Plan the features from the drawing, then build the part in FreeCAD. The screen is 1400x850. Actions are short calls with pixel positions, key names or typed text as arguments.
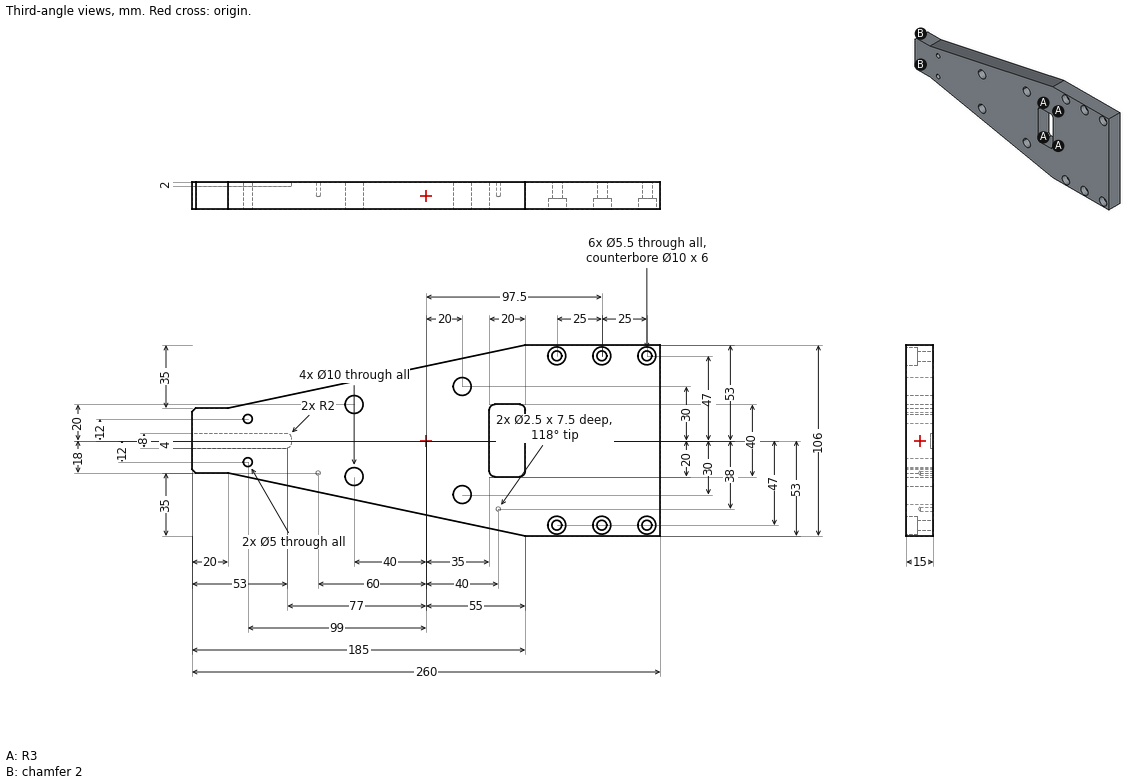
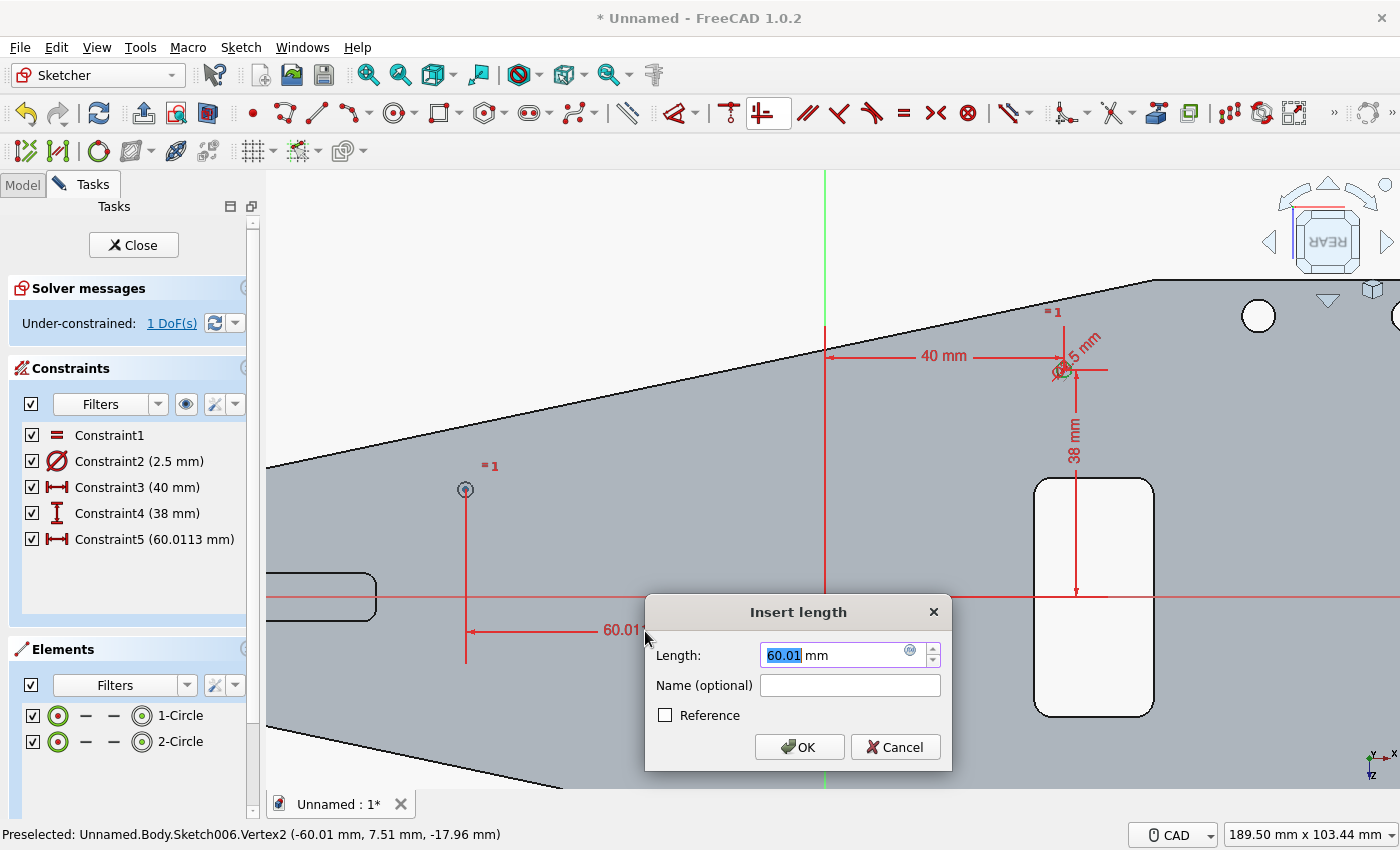
text(60)
key(Return)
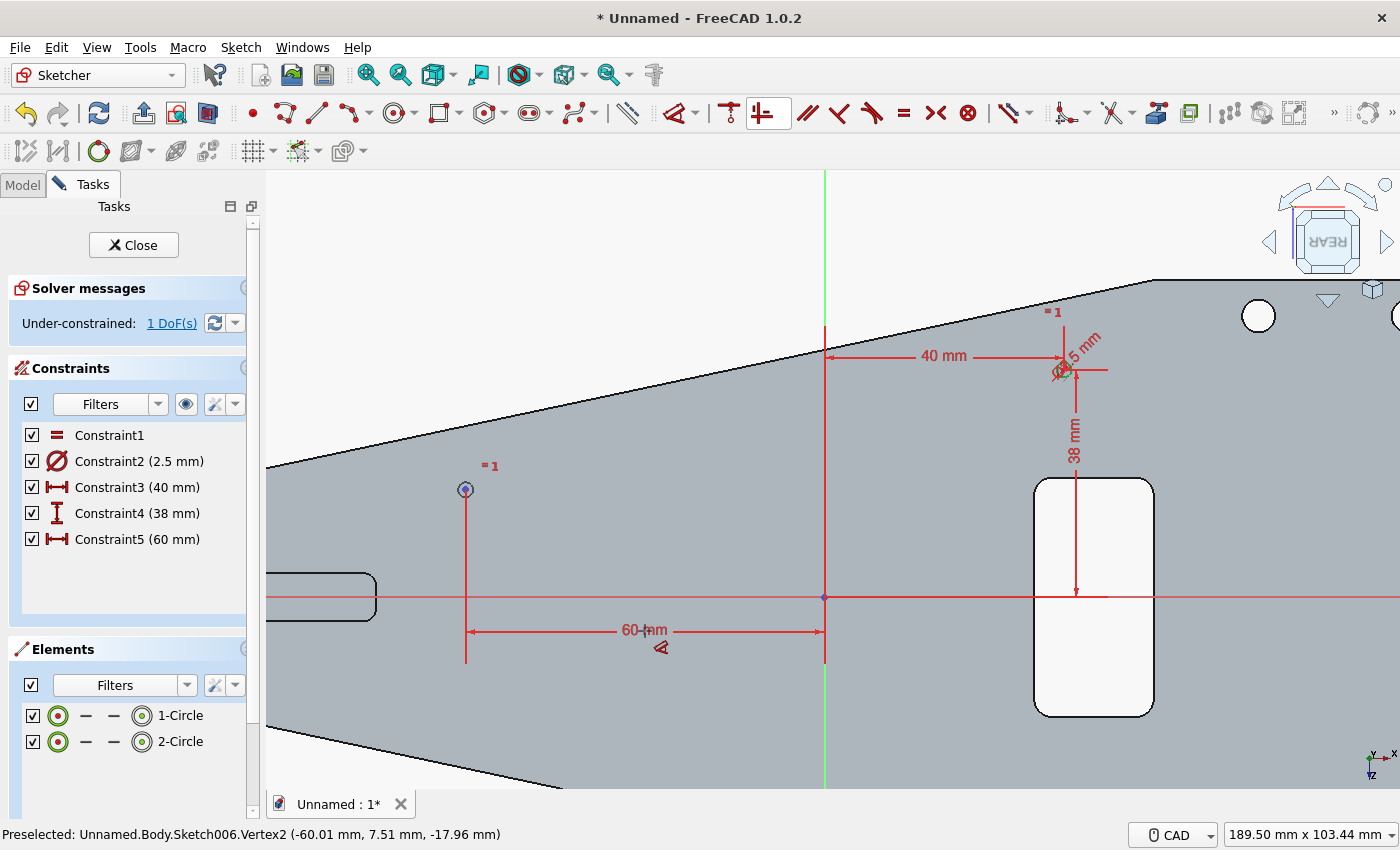
click(466, 490)
click(432, 543)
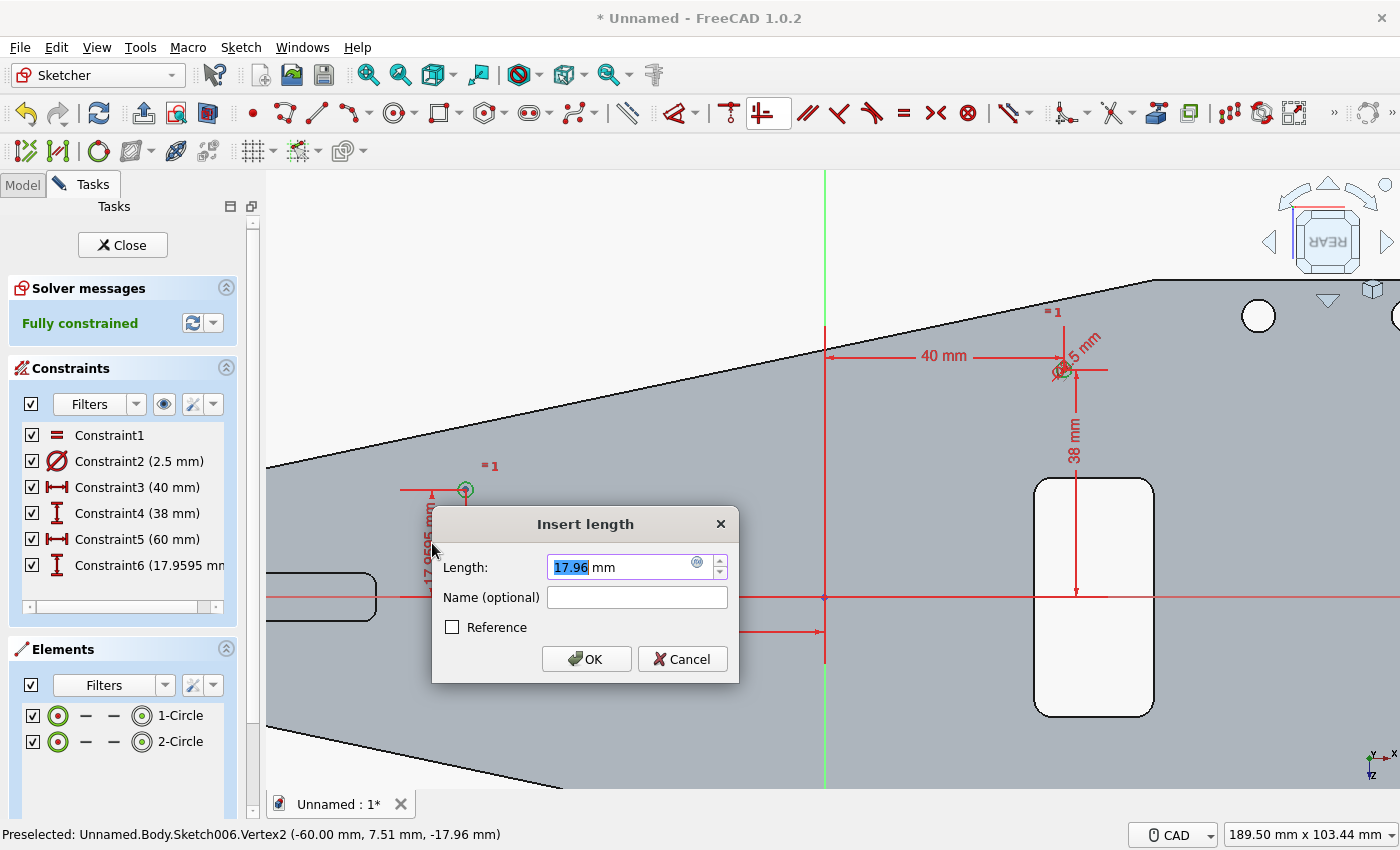
text(18)
key(Return)
key(Escape)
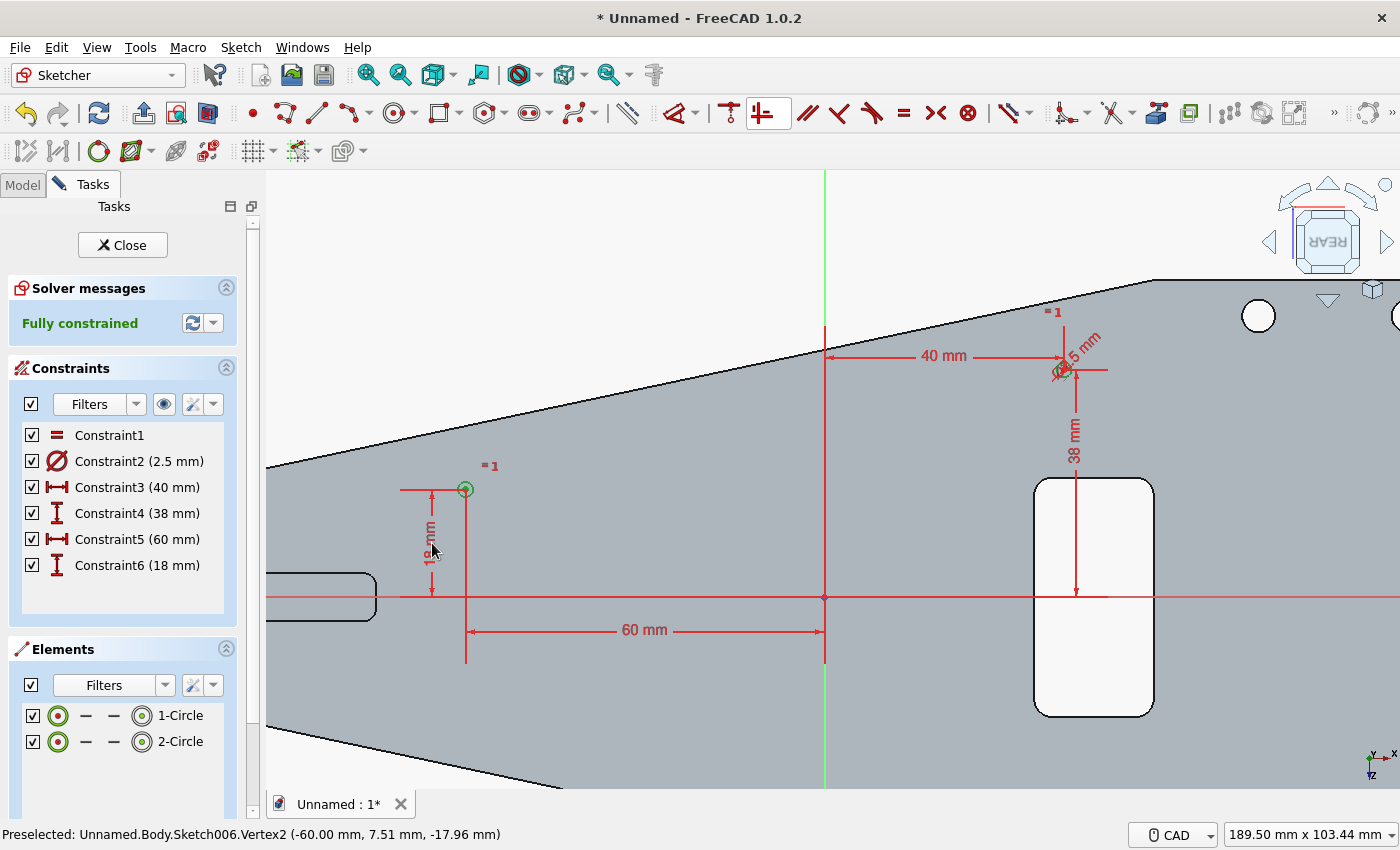
click(123, 245)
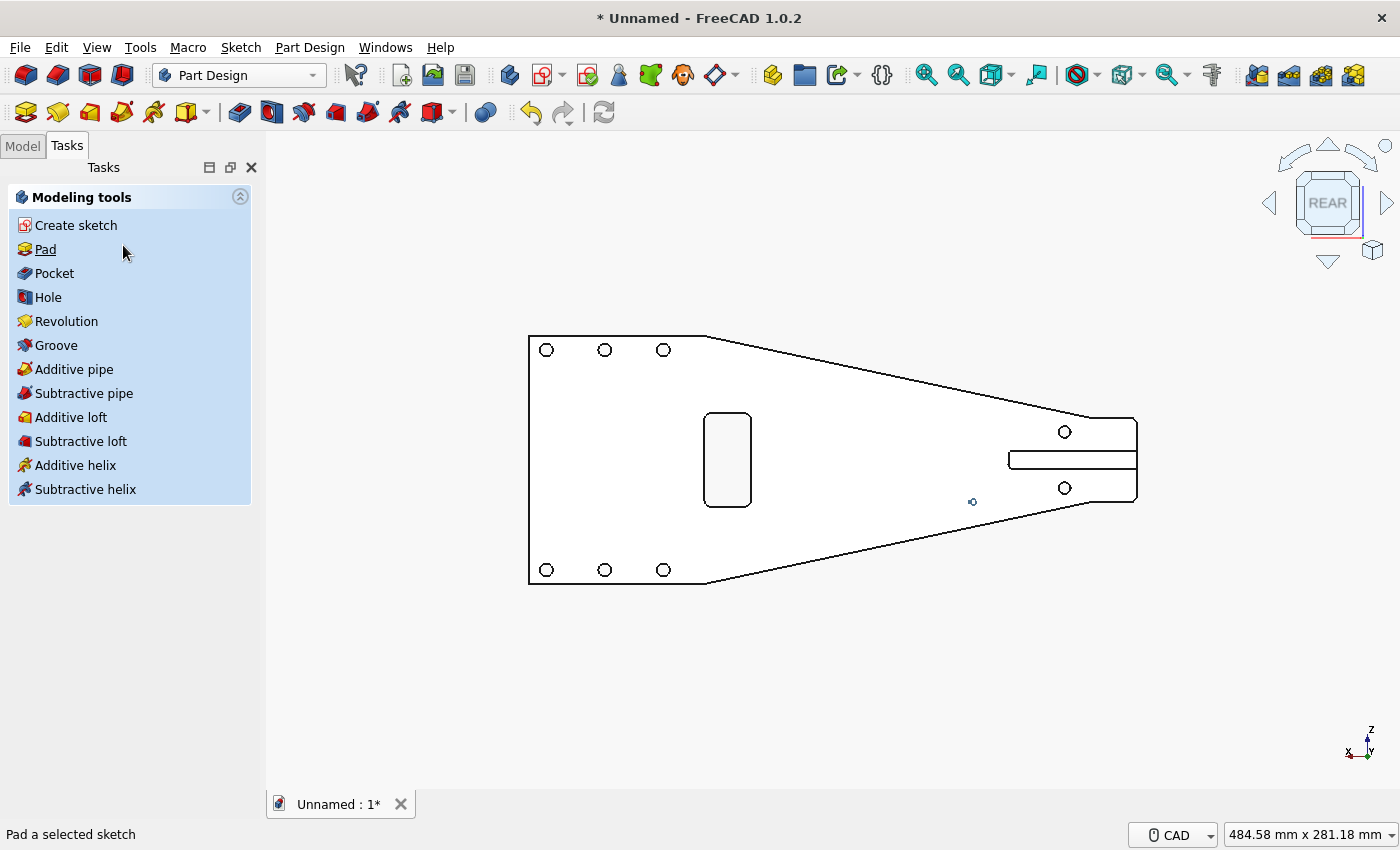
click(272, 112)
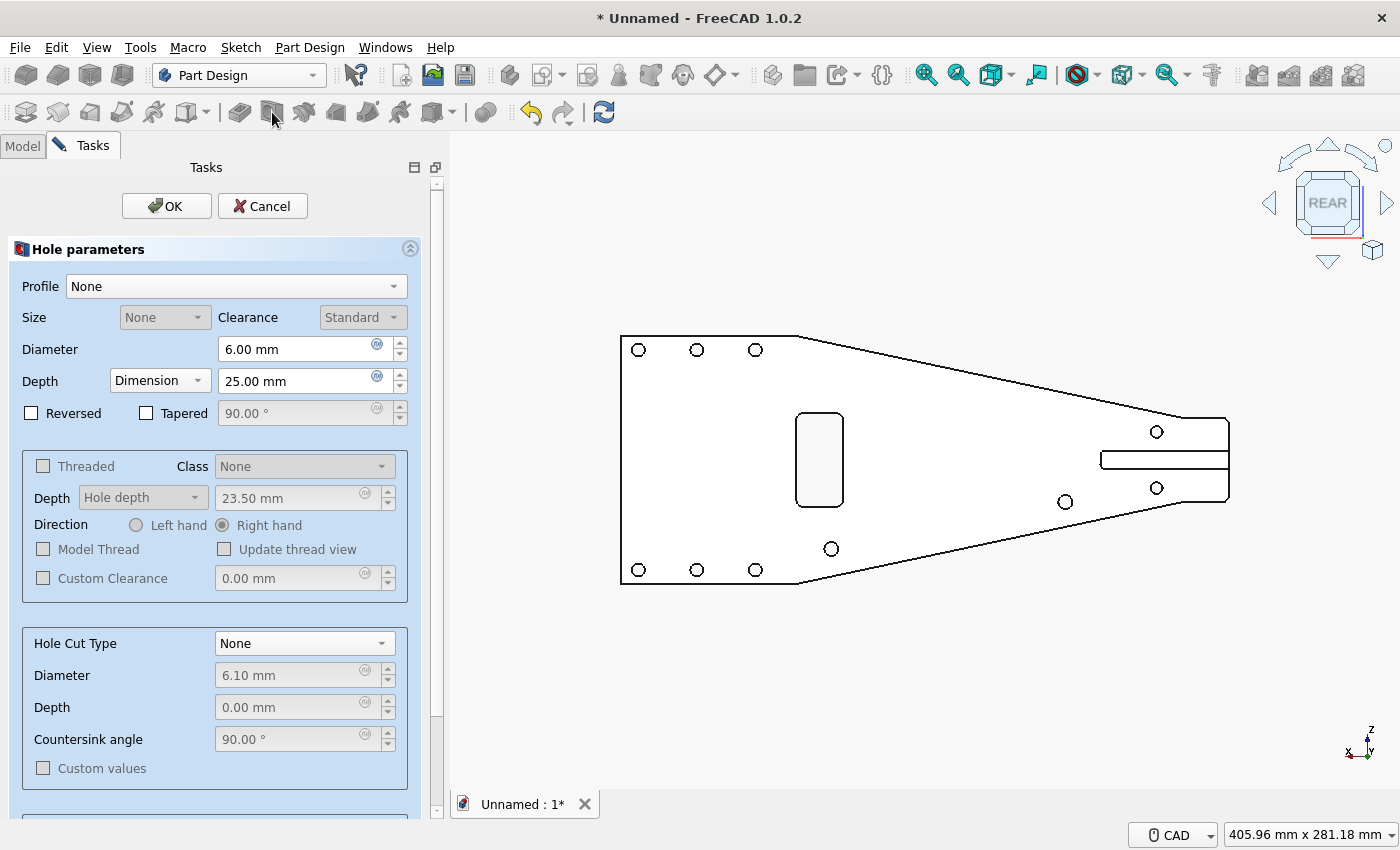
triple_click(305, 349)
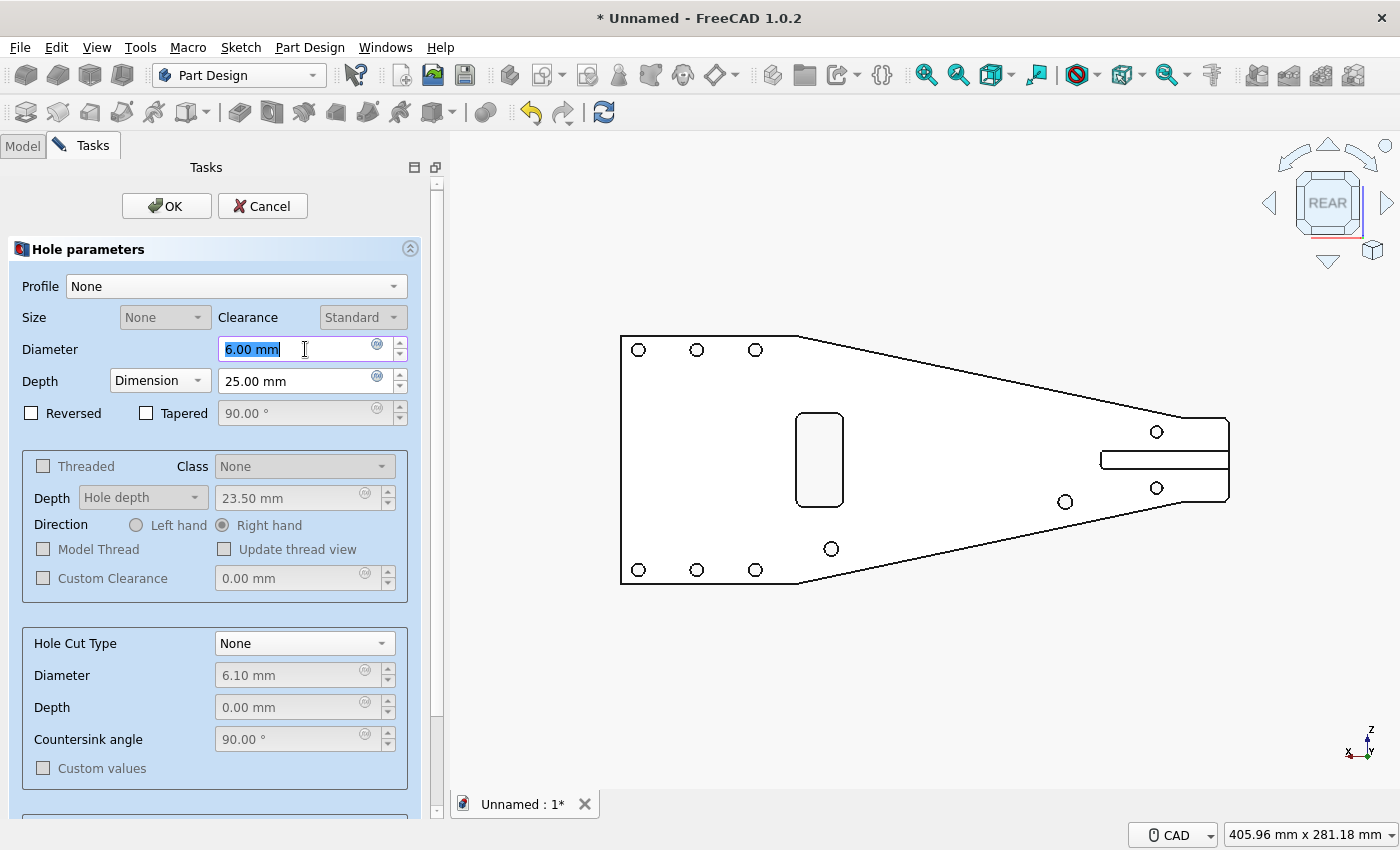
text(2.5)
key(Tab)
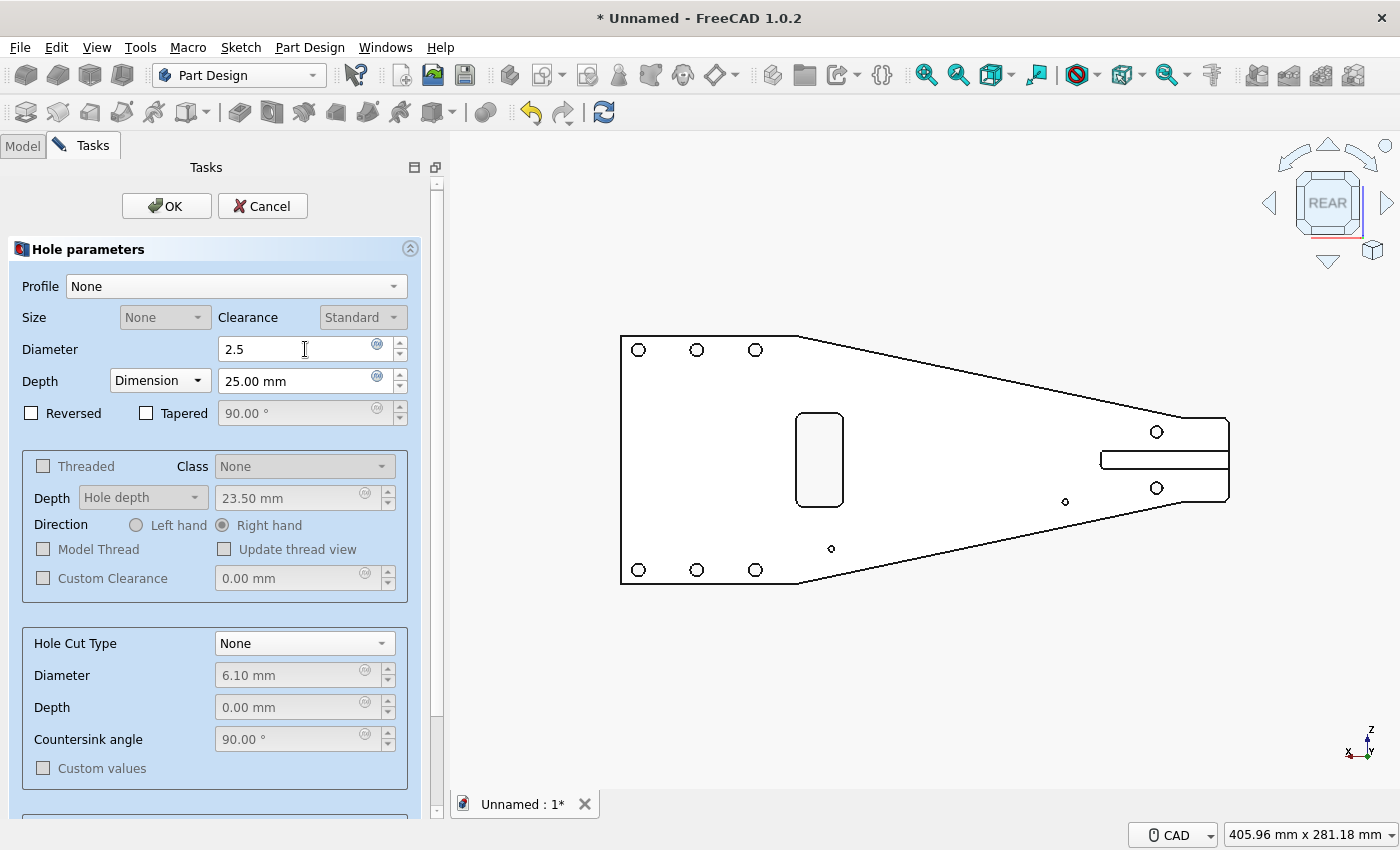
triple_click(305, 381)